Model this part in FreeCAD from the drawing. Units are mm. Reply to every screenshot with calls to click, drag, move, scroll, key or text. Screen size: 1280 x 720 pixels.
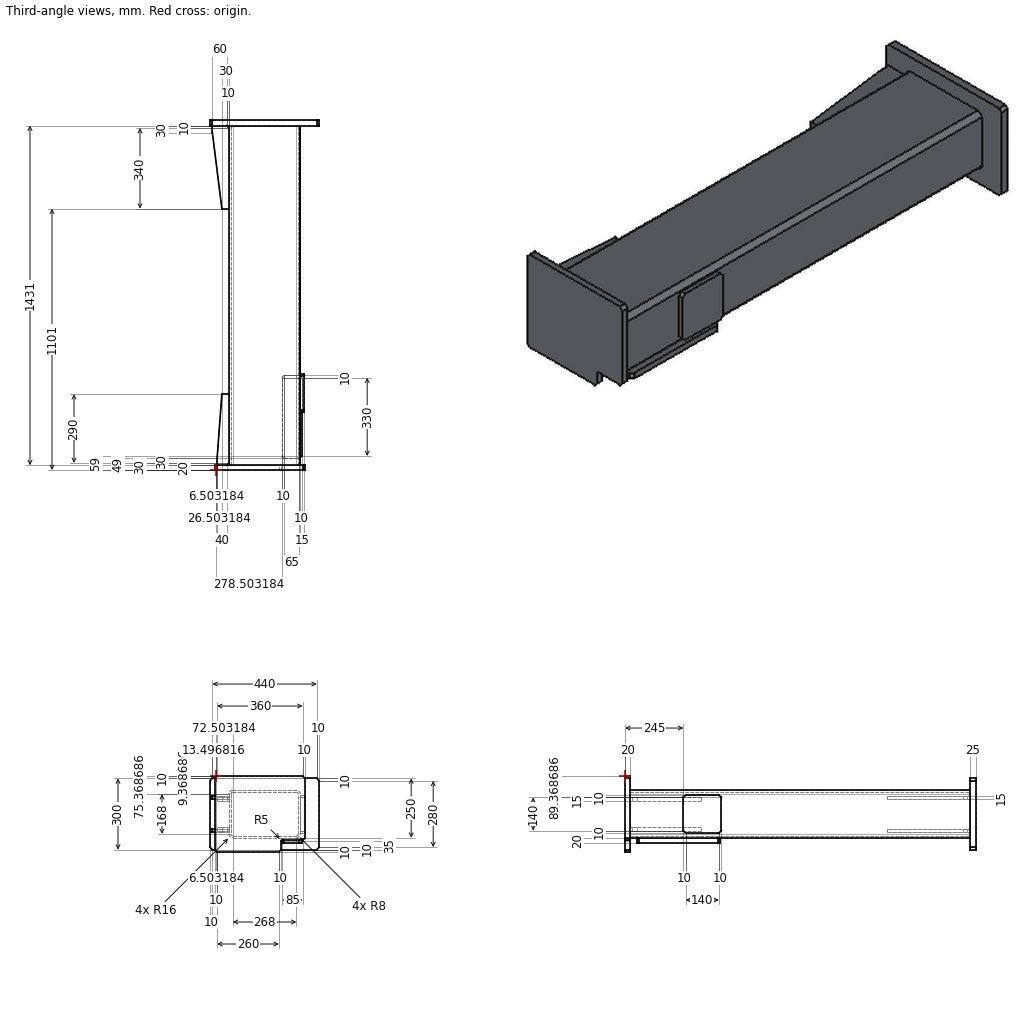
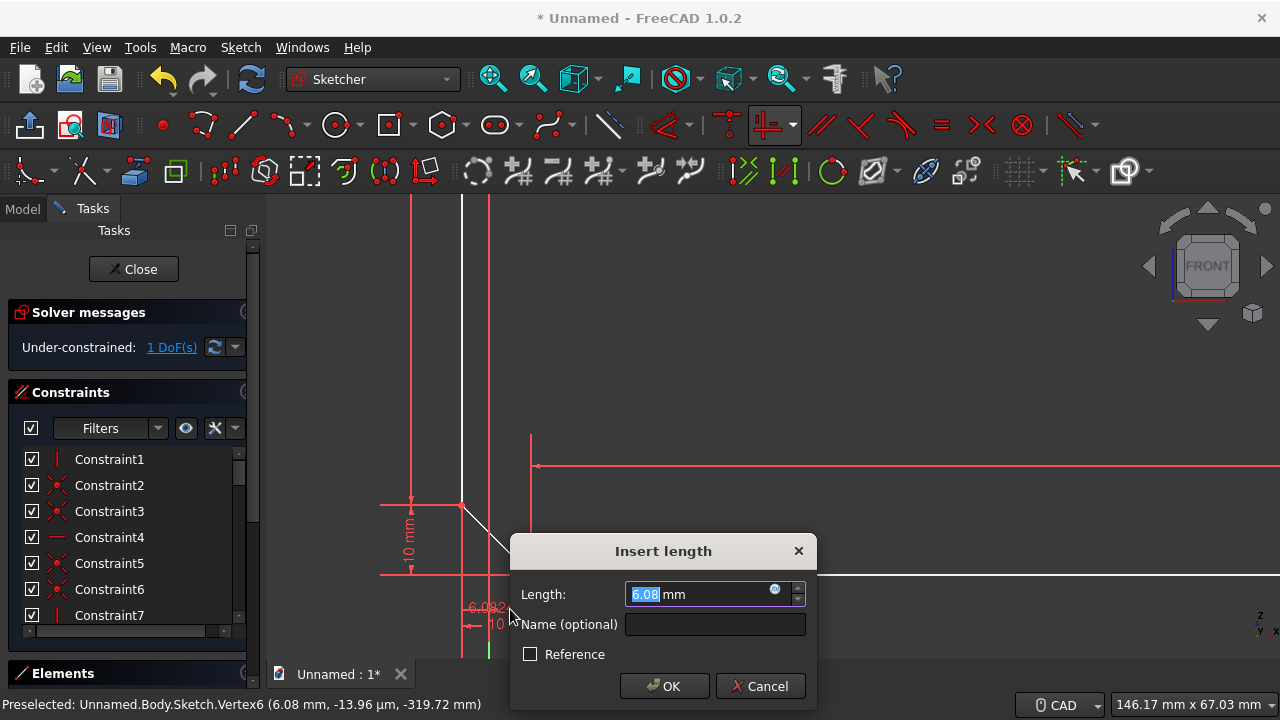
text(6.503184)
key(Return)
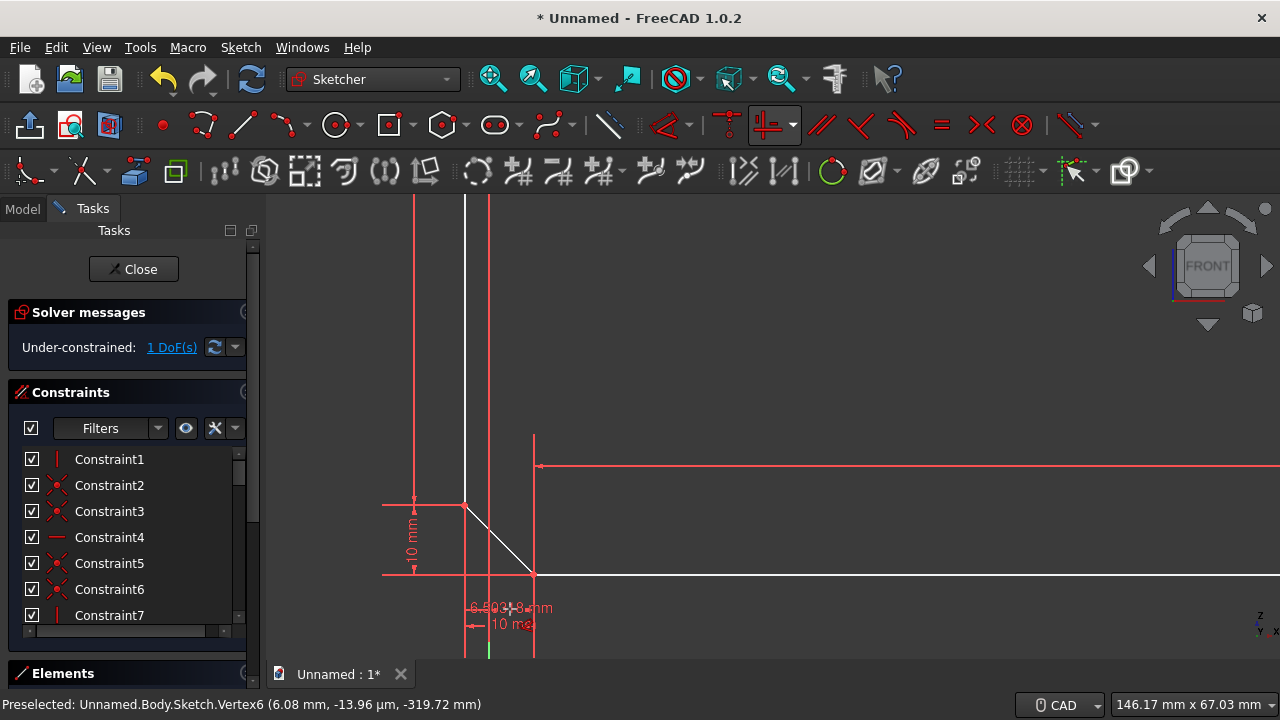
scroll(536, 577, down, 10)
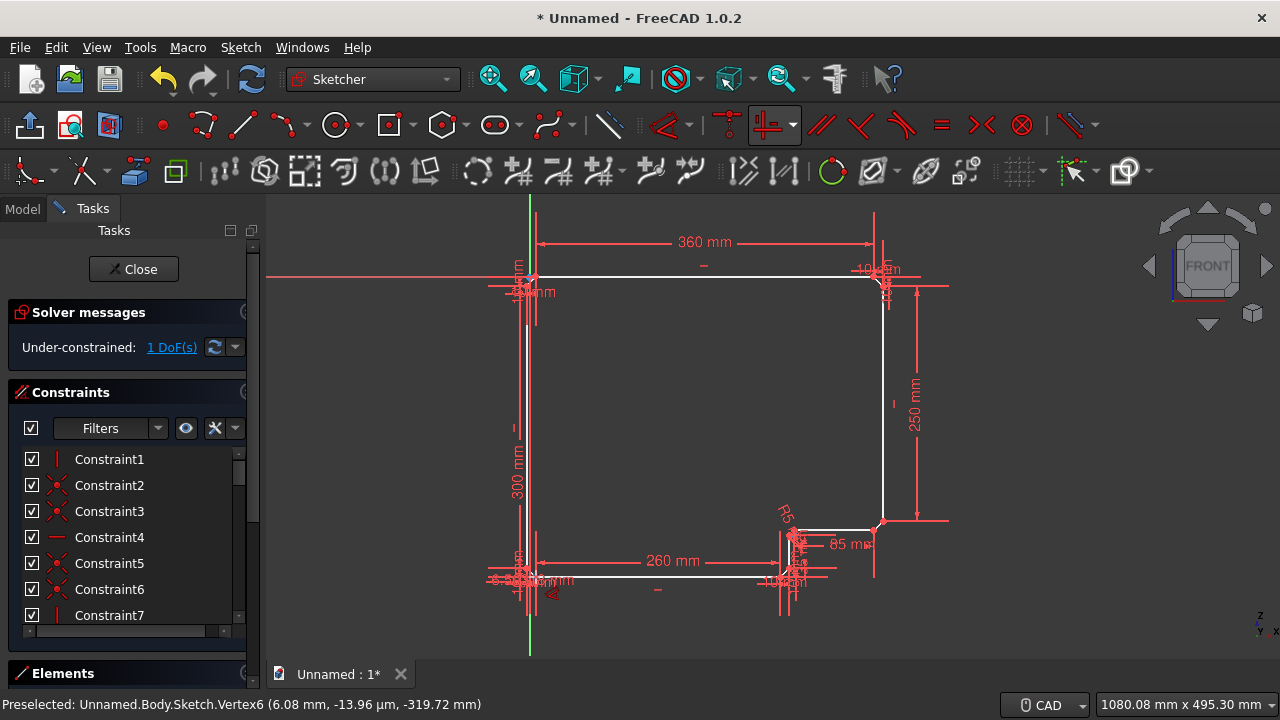
scroll(527, 286, up, 8)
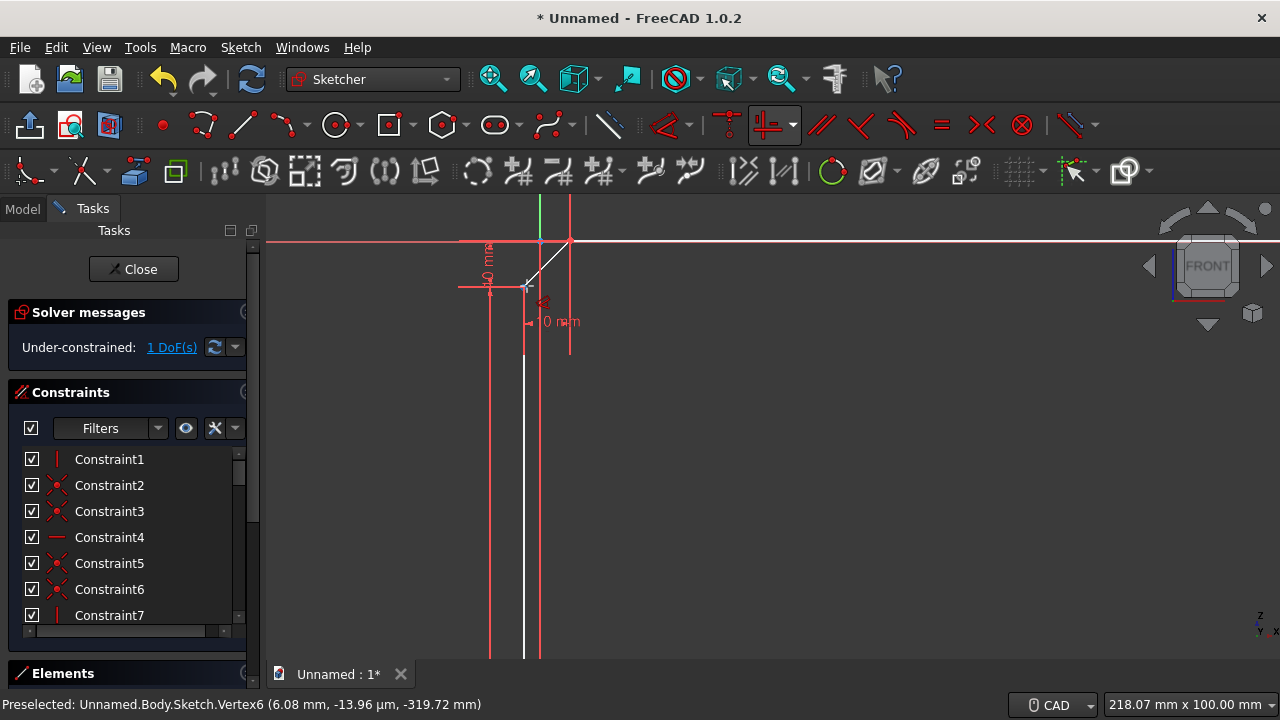
click(524, 287)
click(574, 264)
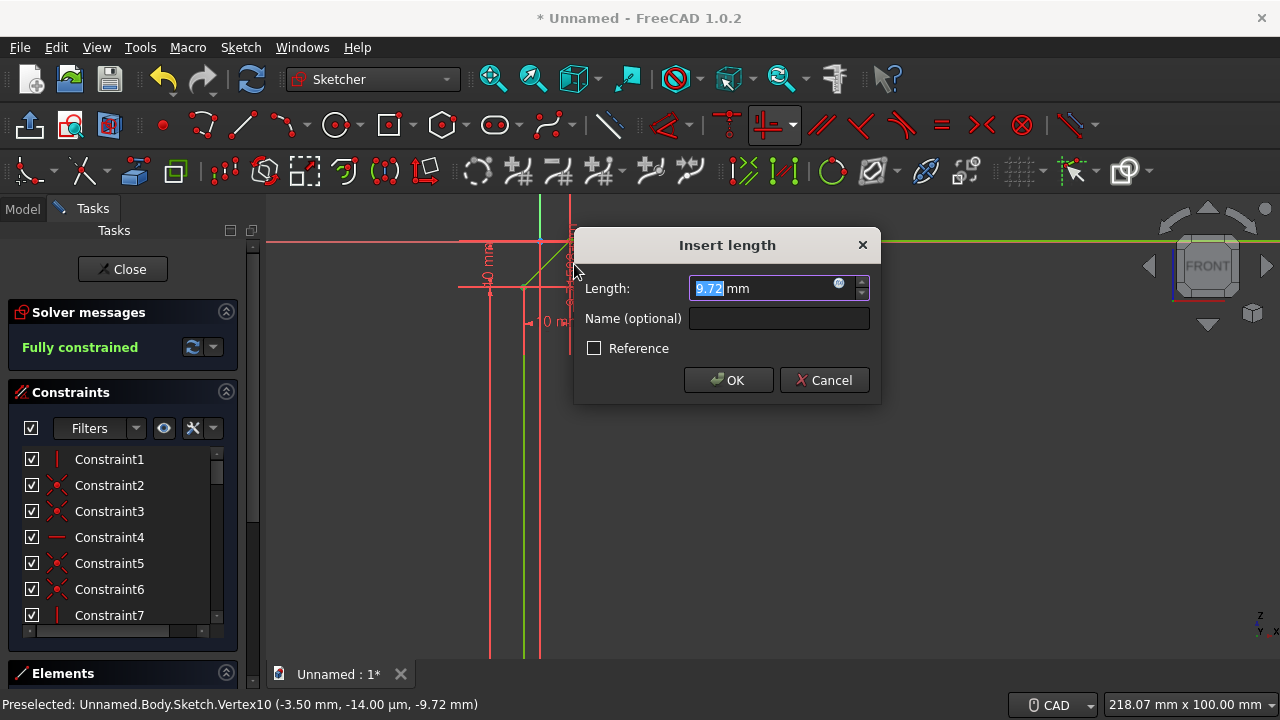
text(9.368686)
key(Return)
key(Escape)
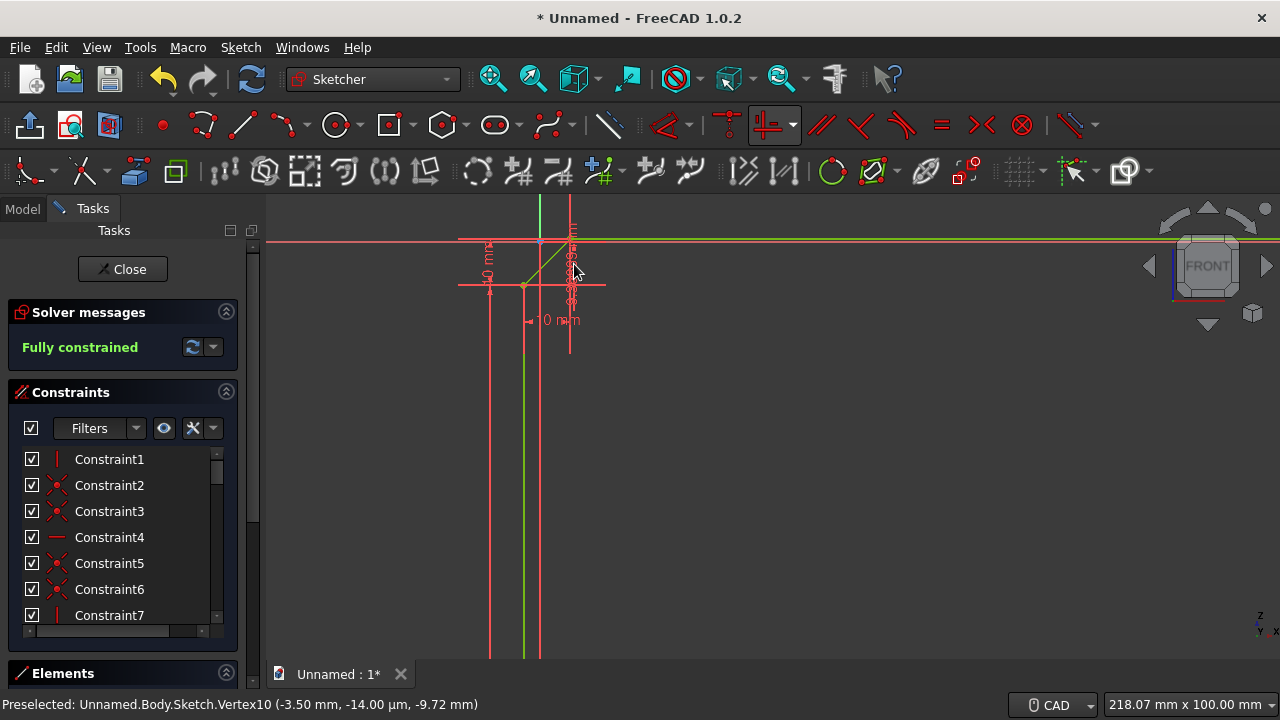
click(123, 269)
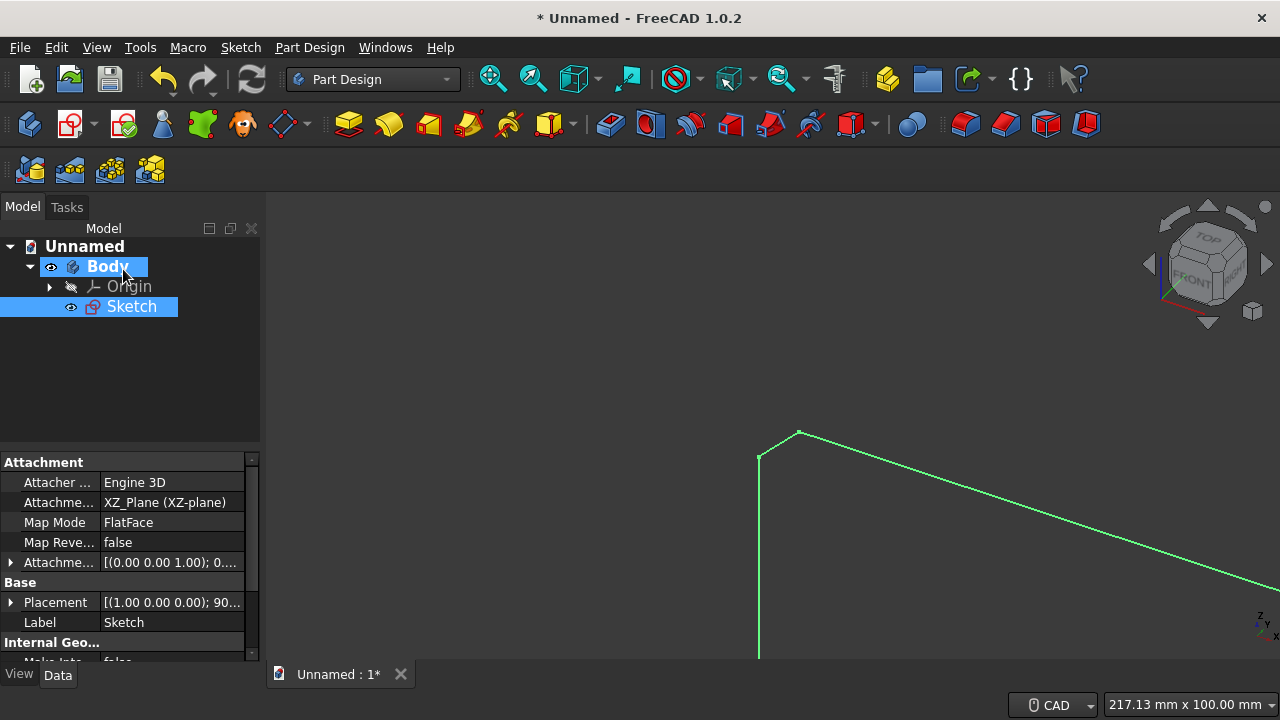
click(350, 124)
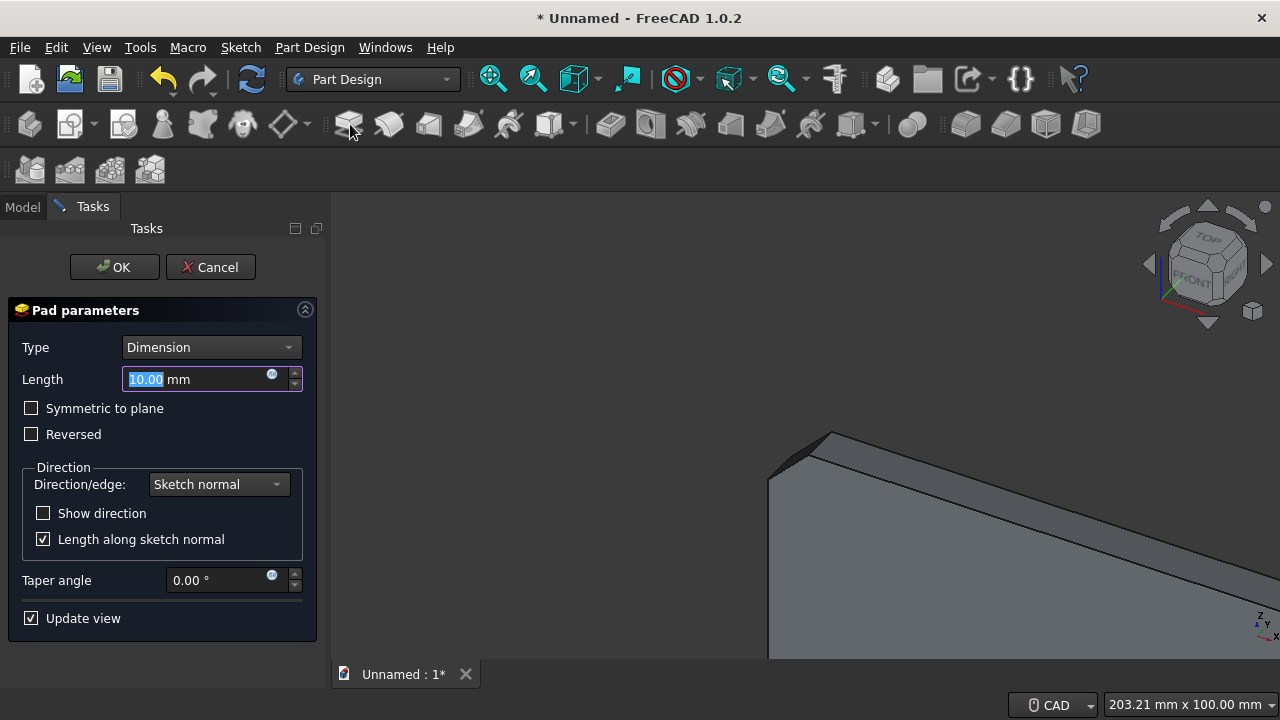
text(20)
key(Tab)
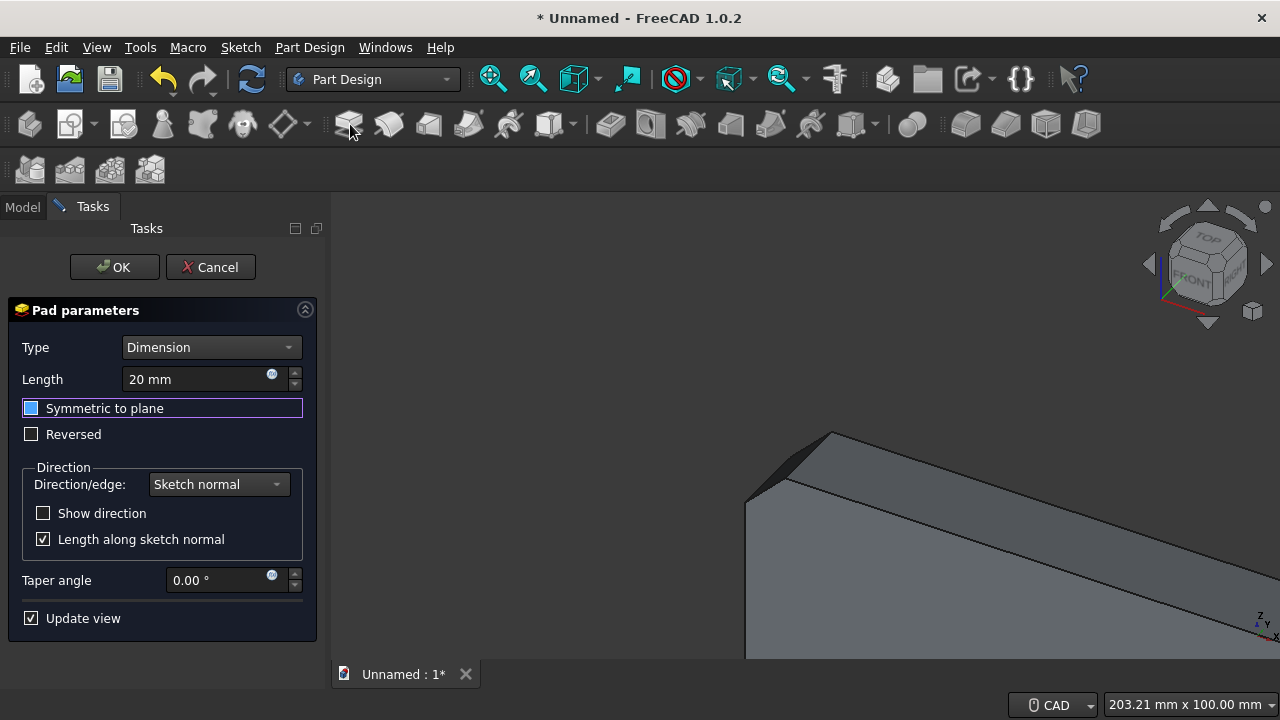
click(30, 434)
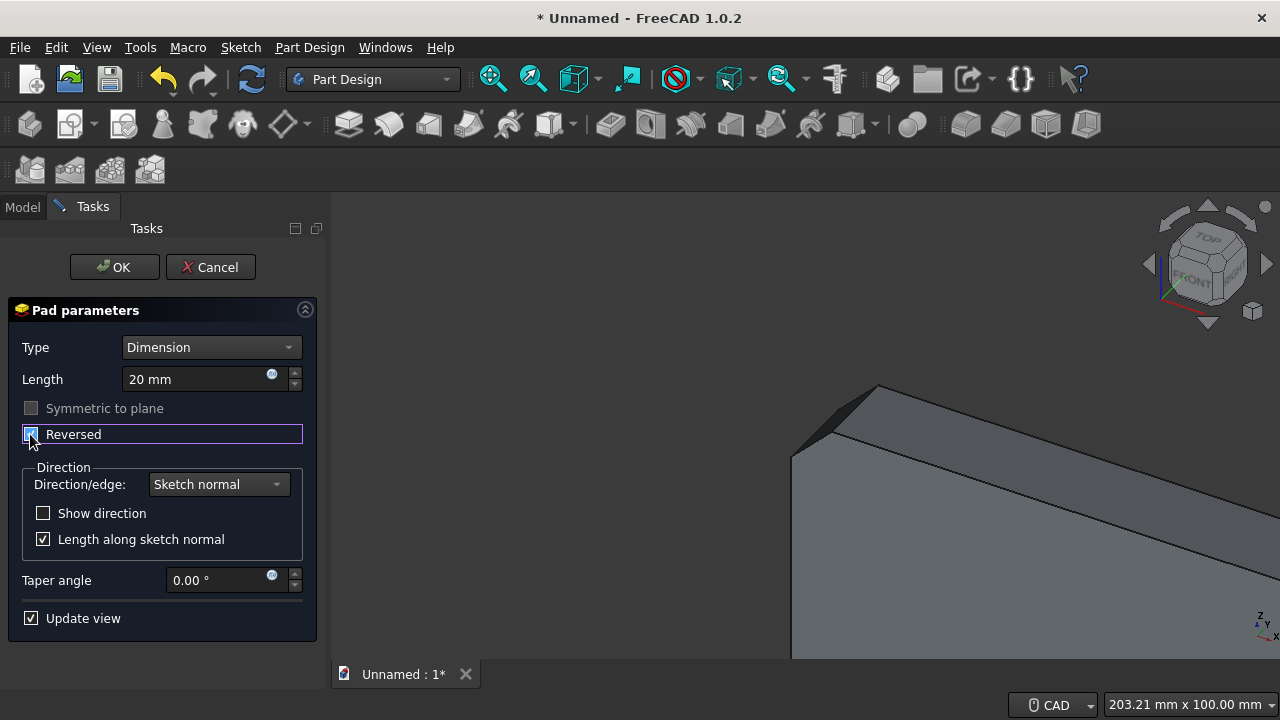
click(115, 267)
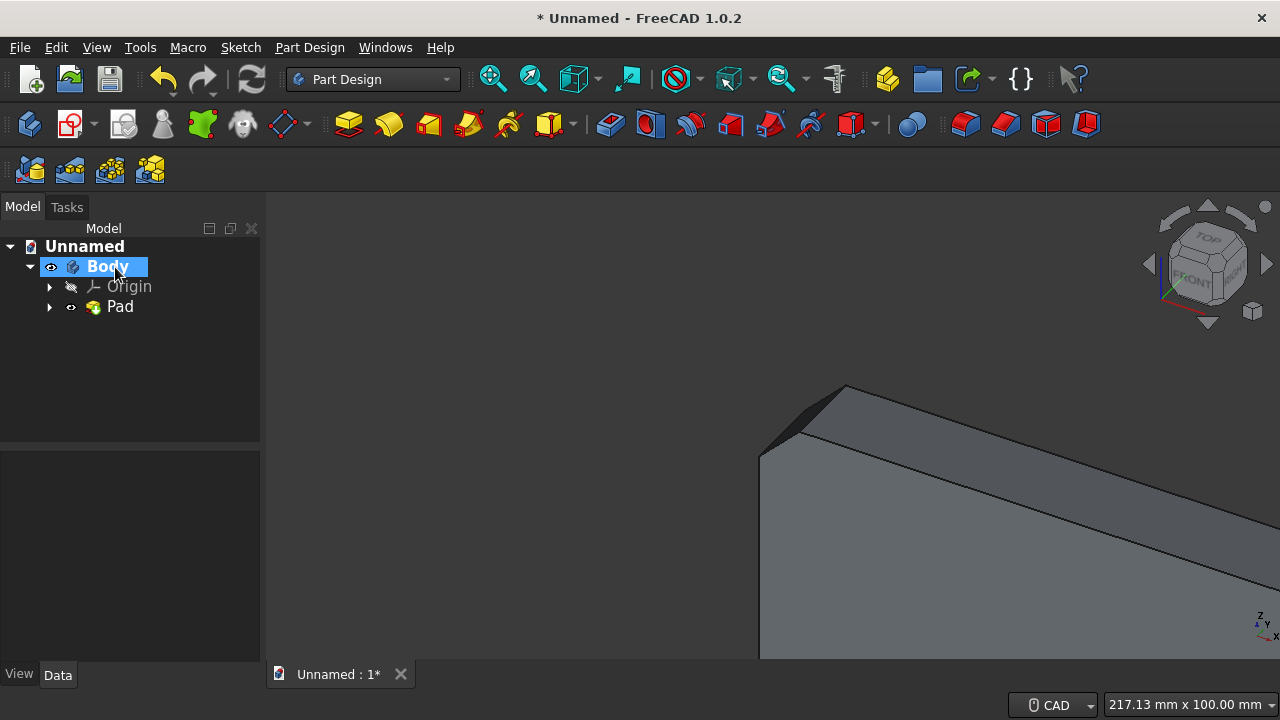
key(v)
key(f)